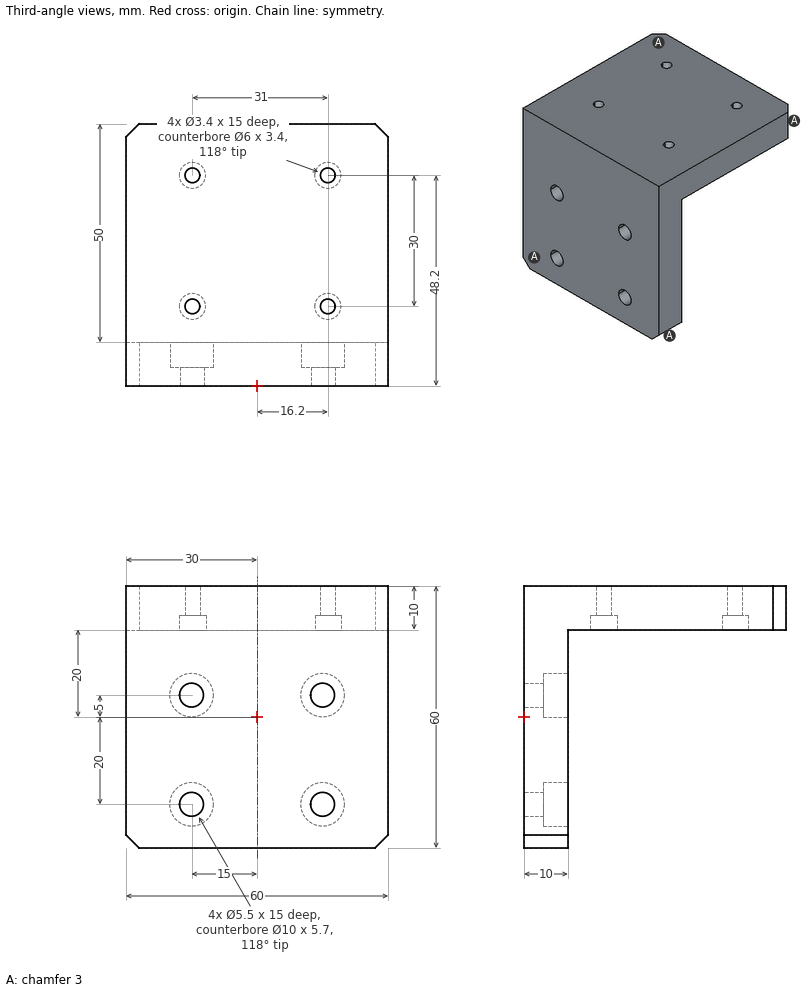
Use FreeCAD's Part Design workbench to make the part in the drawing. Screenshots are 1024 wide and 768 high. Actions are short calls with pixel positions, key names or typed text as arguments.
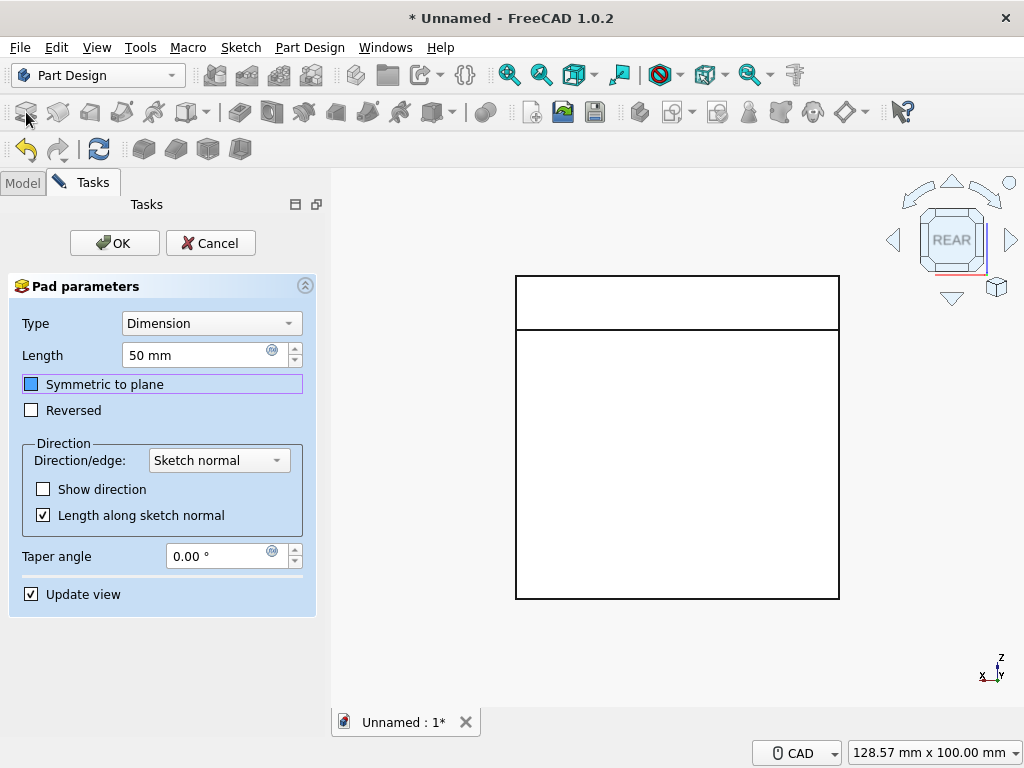
click(115, 243)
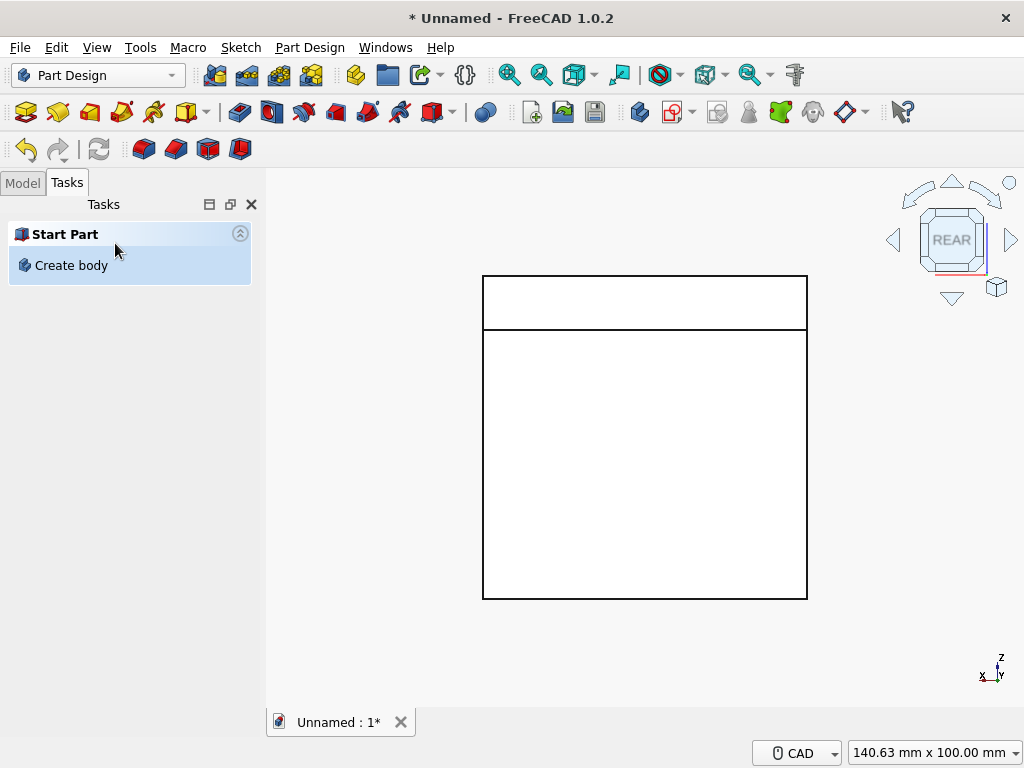
click(807, 302)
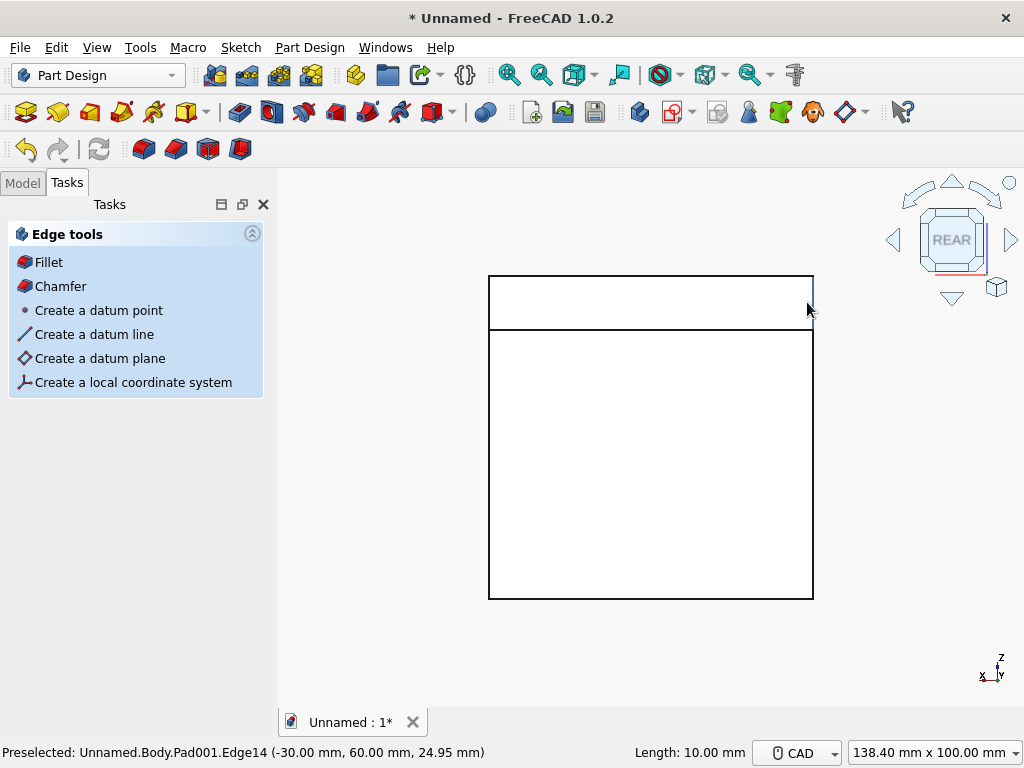
key(0)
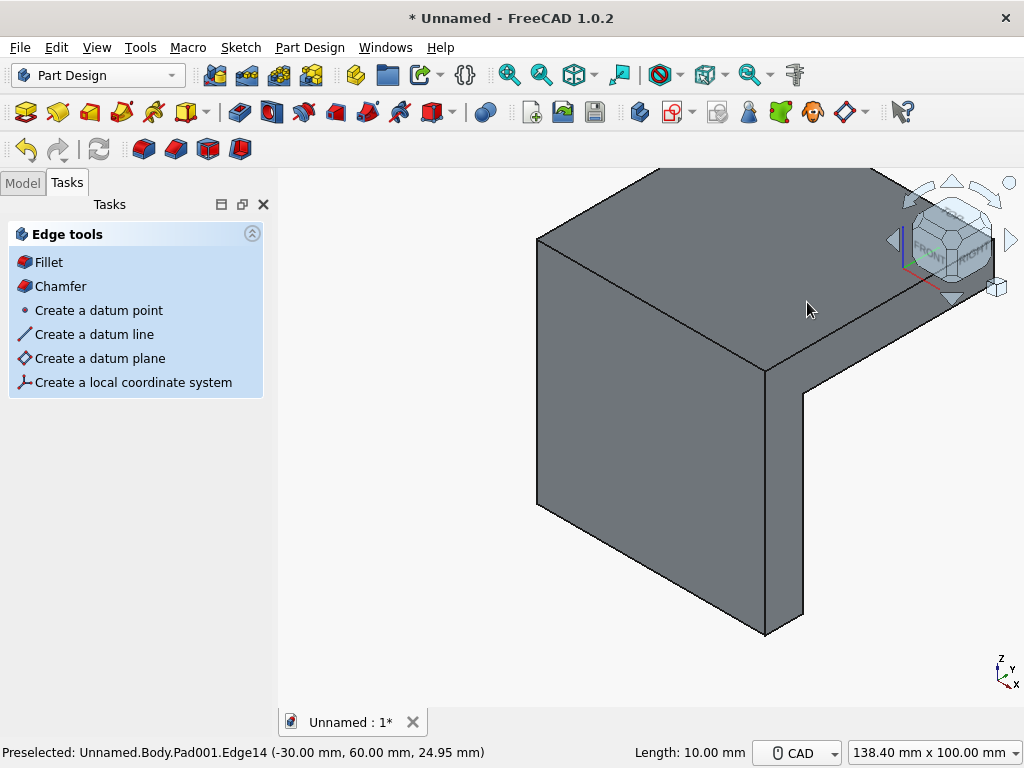
click(510, 76)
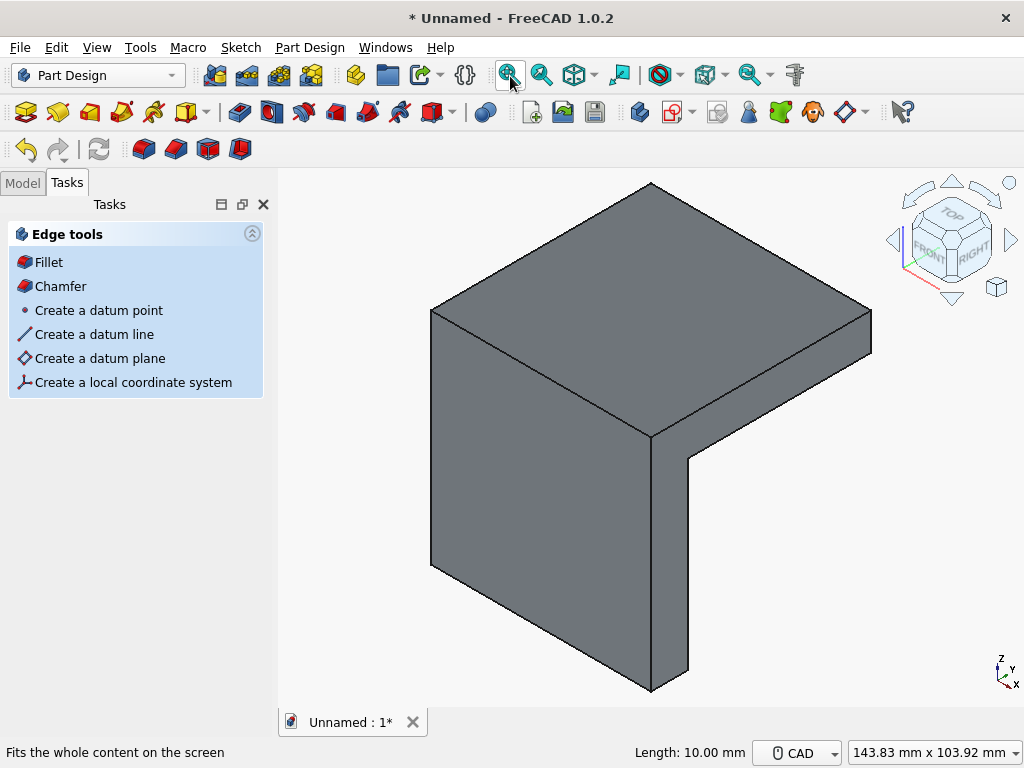
key(2)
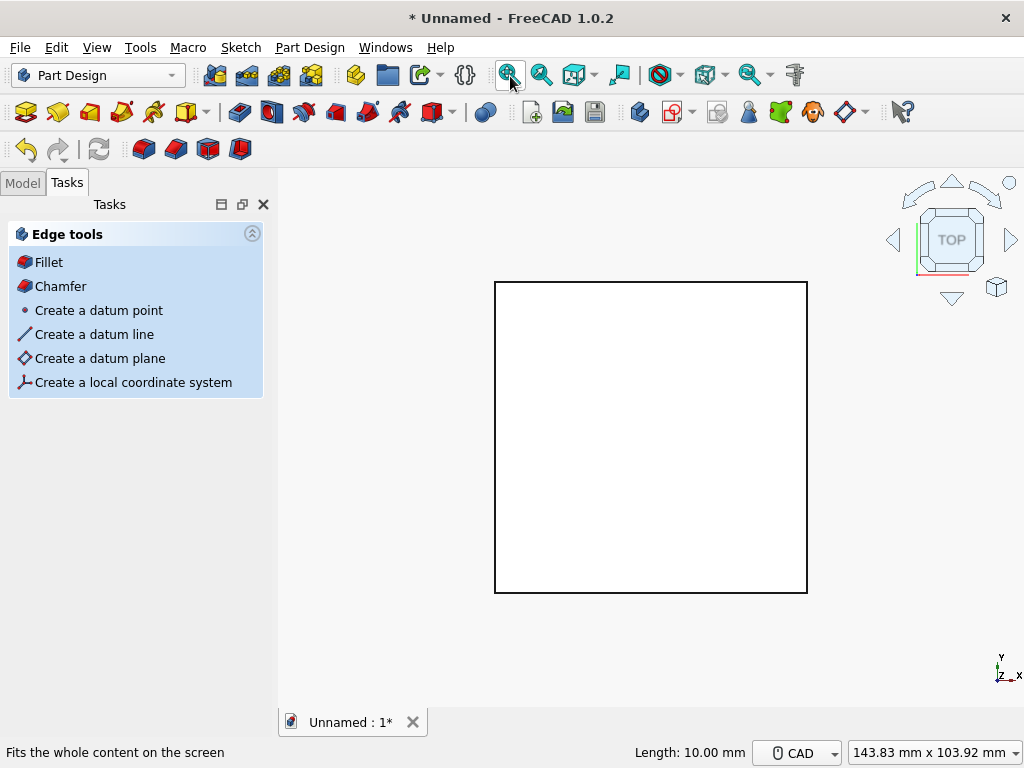
key(1)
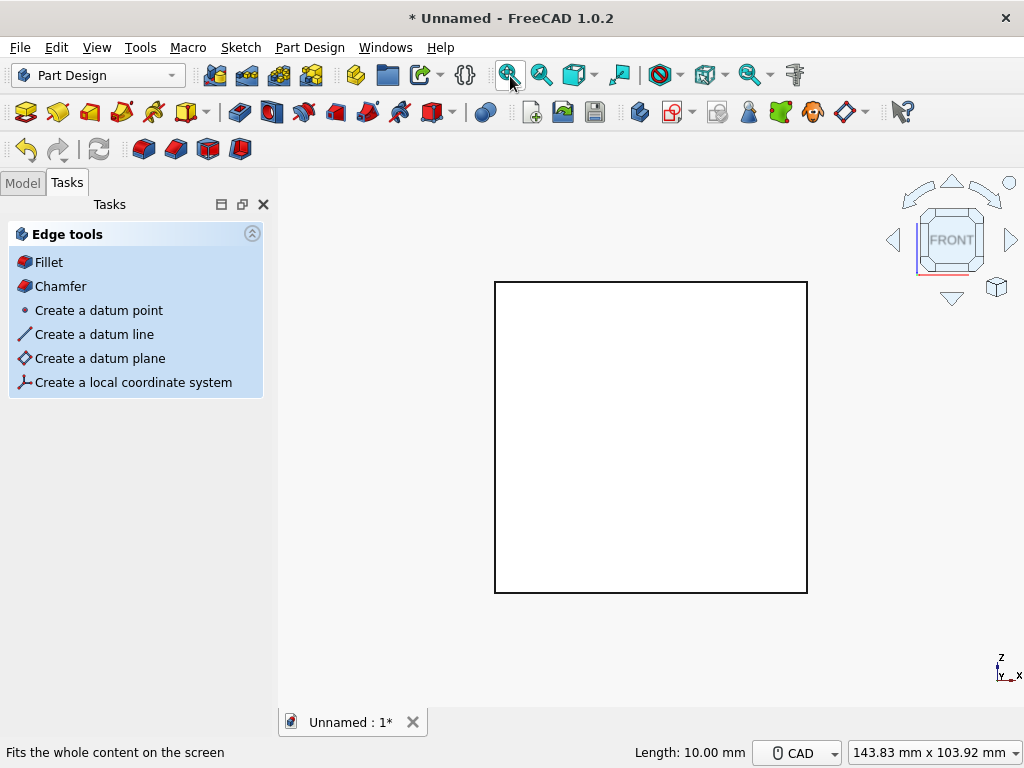
key(3)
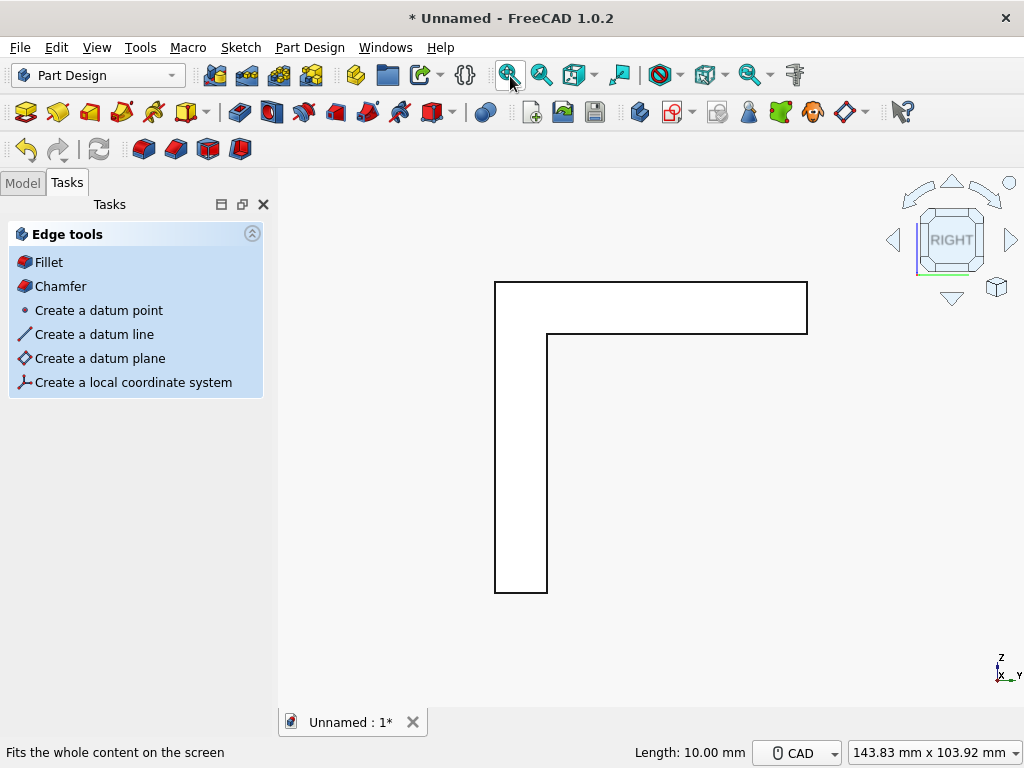
click(807, 307, ctrl)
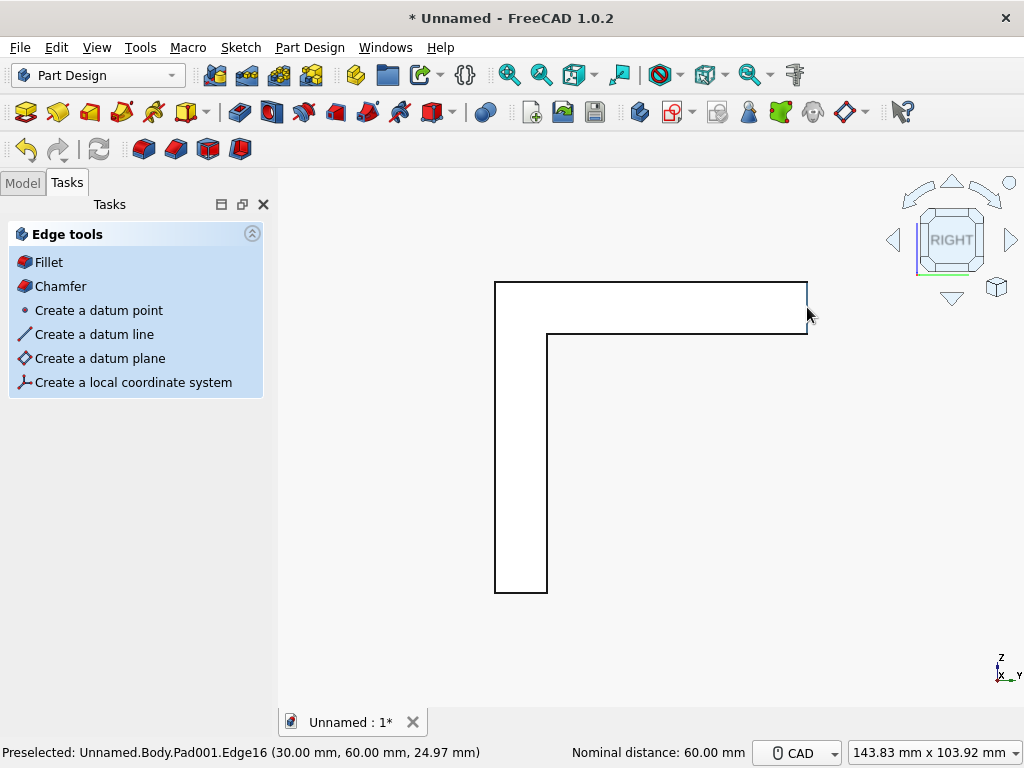
click(521, 592, ctrl)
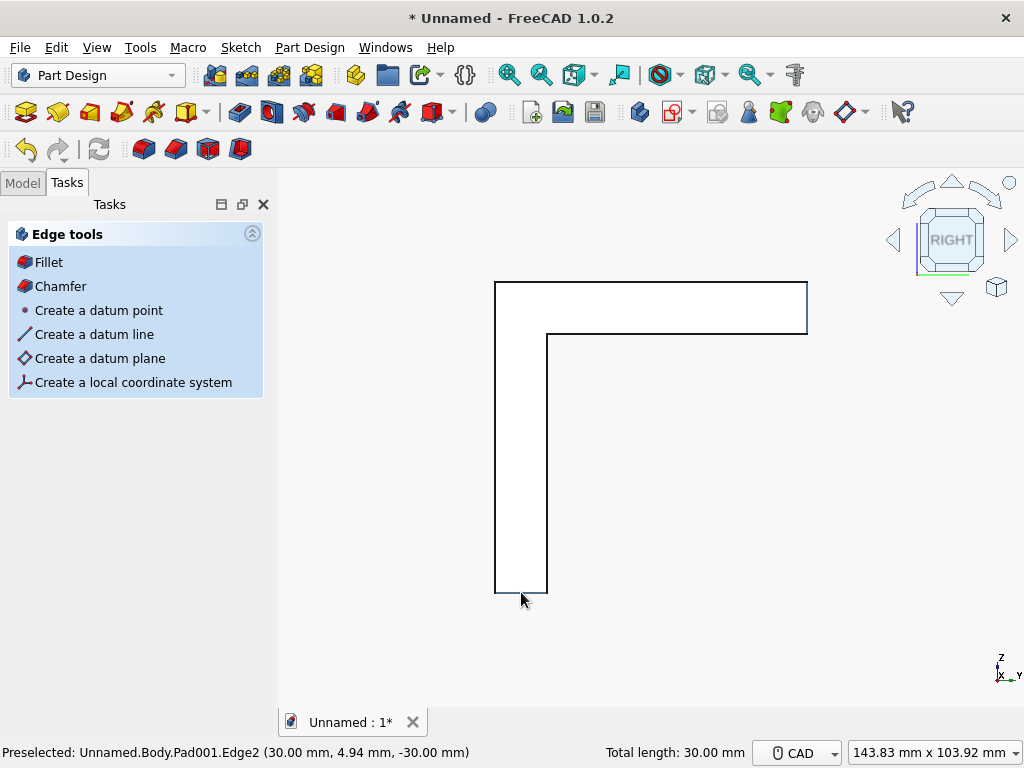
key(5)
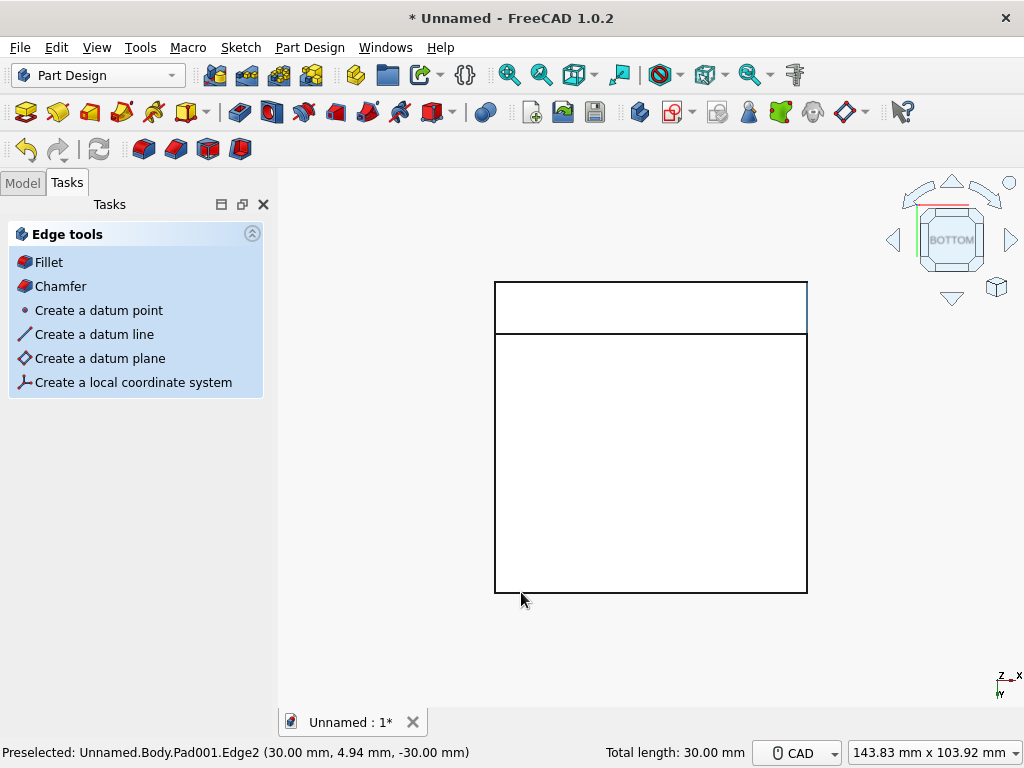
click(495, 307, ctrl)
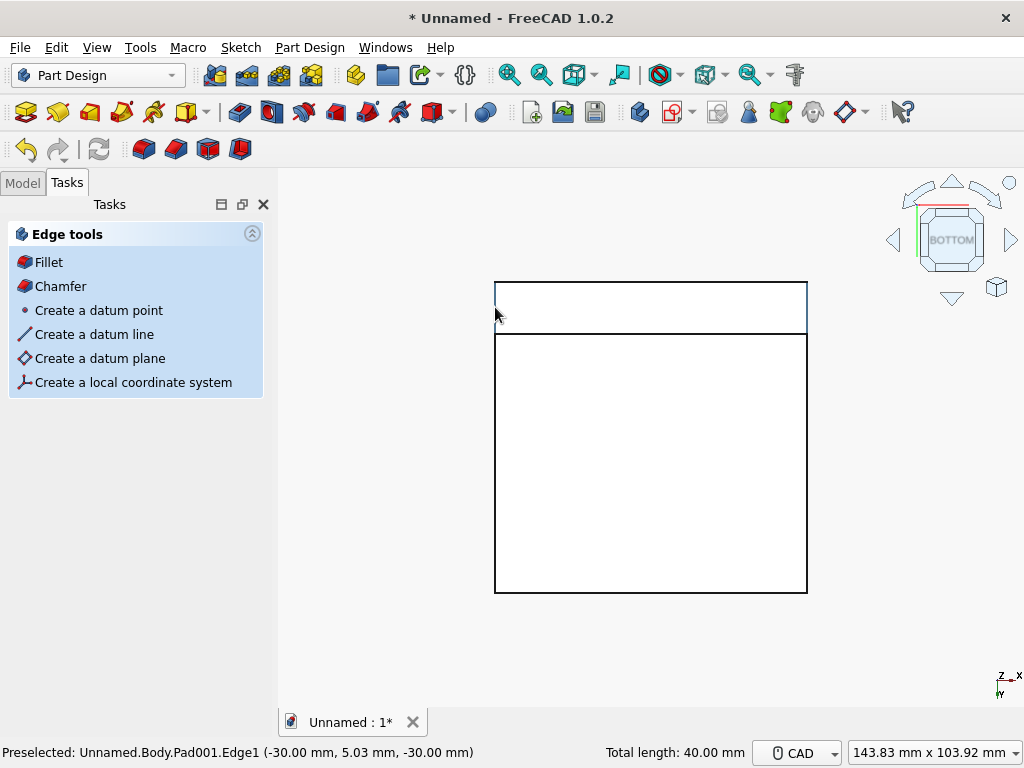
click(176, 150)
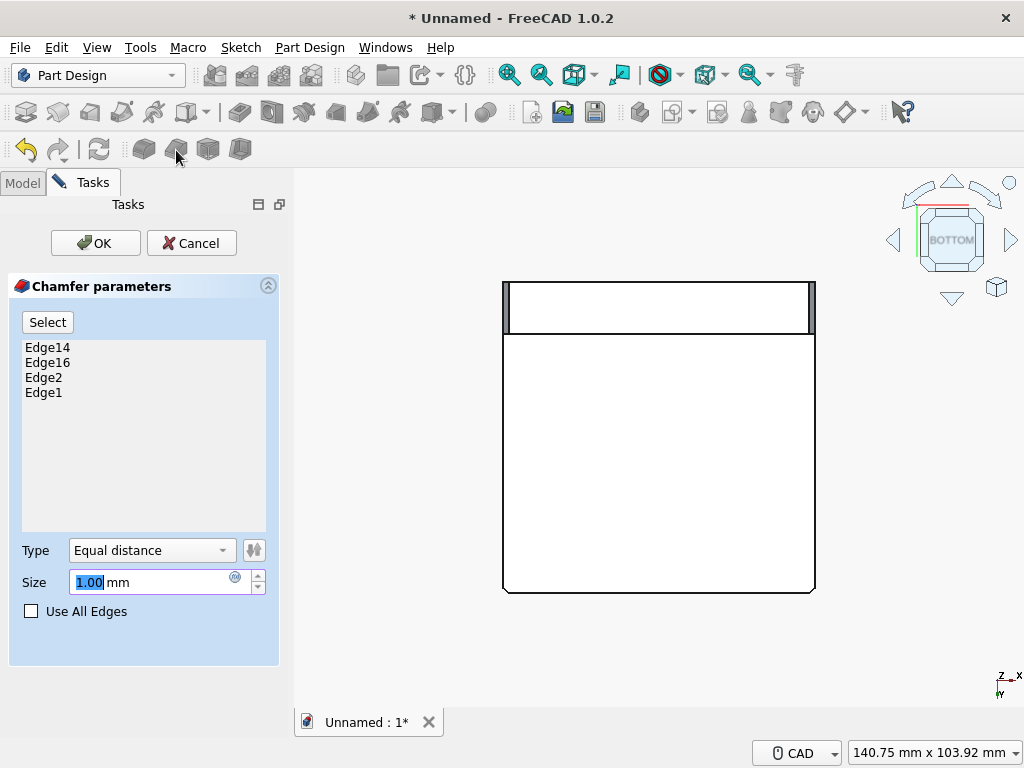
text(3)
key(Tab)